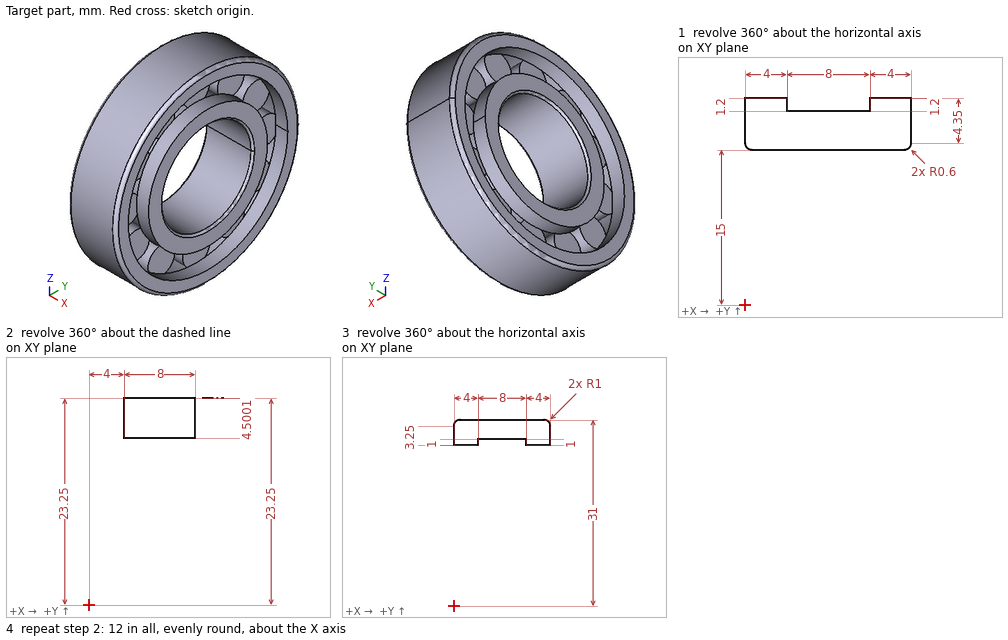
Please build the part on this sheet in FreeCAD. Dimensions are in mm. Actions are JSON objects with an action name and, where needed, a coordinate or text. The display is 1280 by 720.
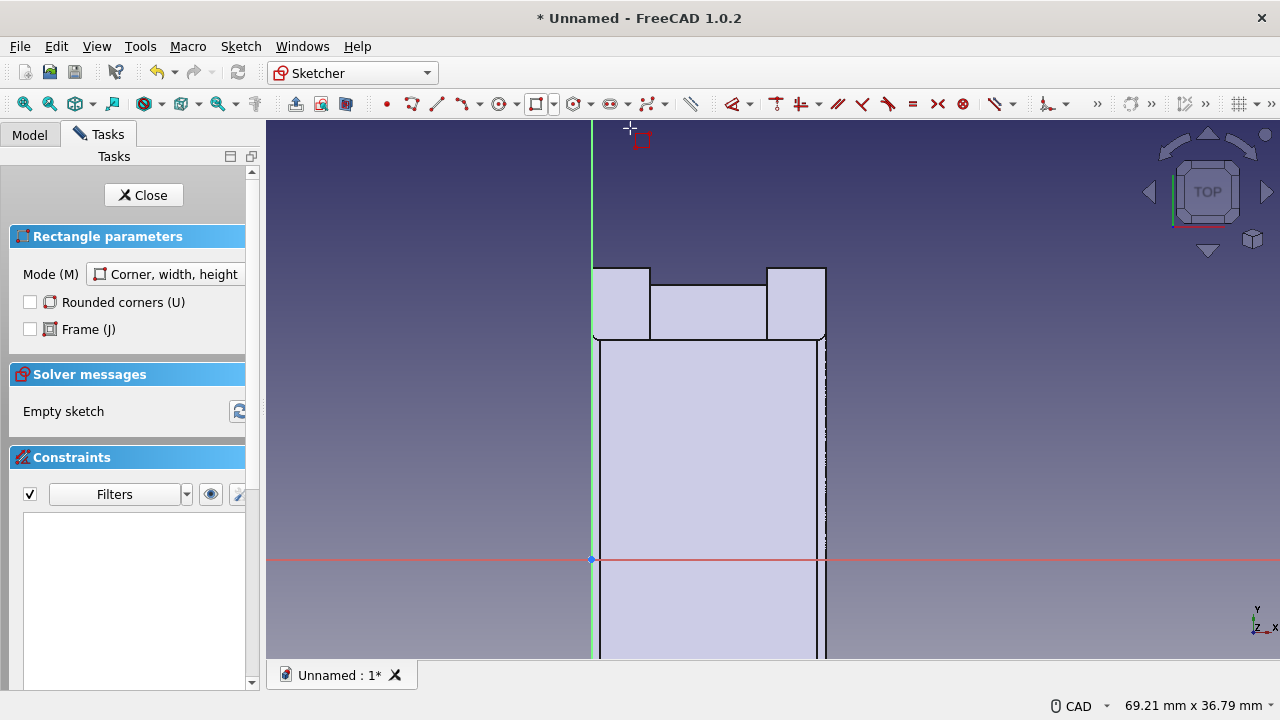
{"action": "left_click", "coordinate": [650, 219]}
{"action": "mouse_move", "coordinate": [767, 285]}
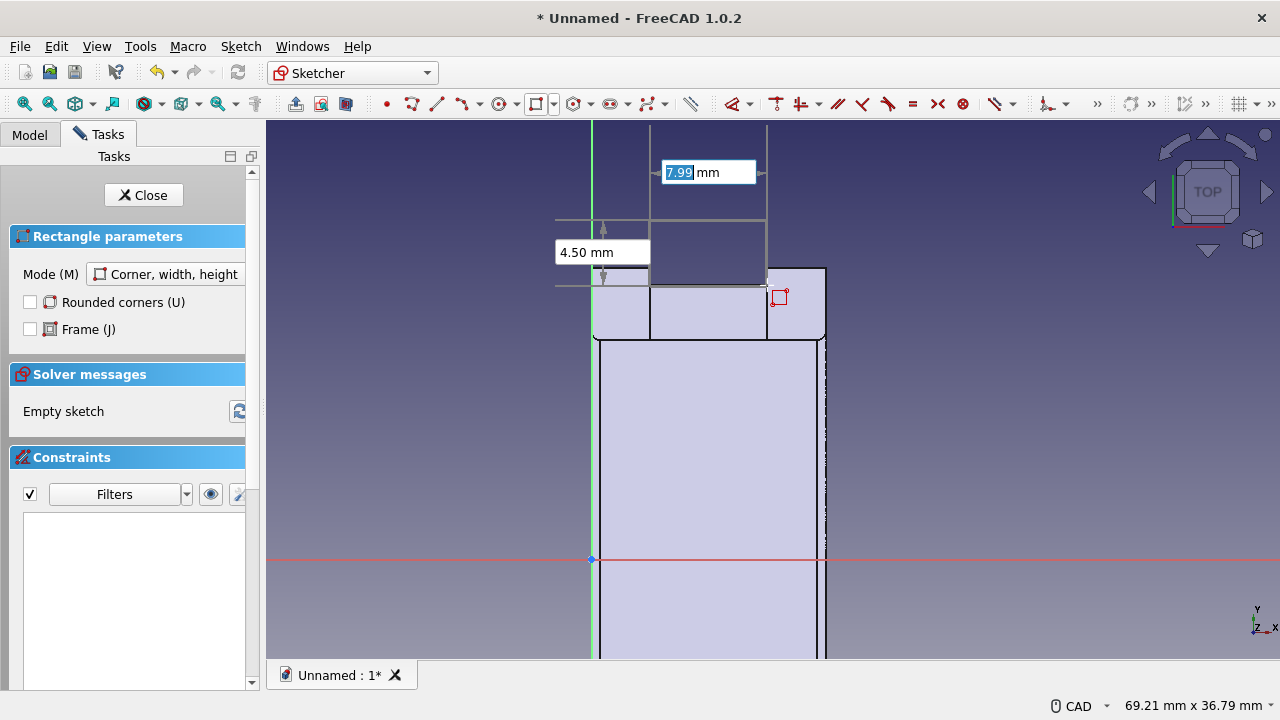
{"action": "type", "text": "8"}
{"action": "key", "text": "Tab"}
{"action": "type", "text": "4.5001"}
{"action": "key", "text": "Return"}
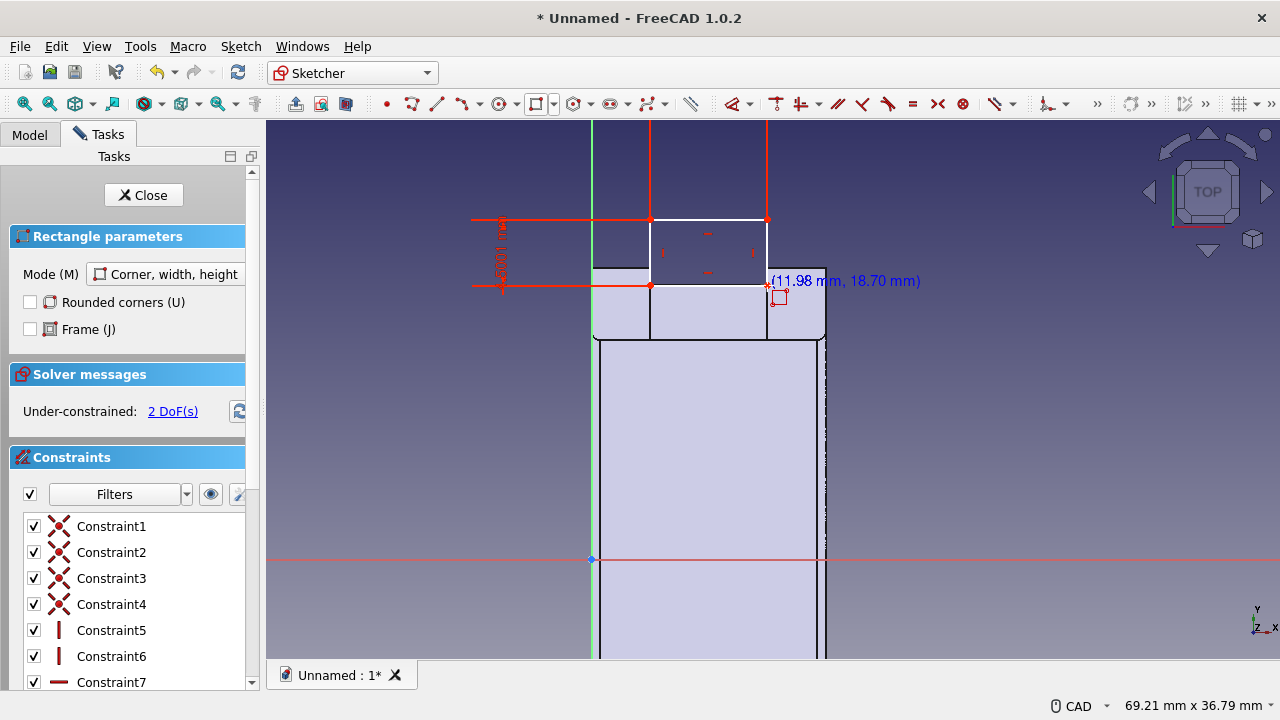
{"action": "left_click", "coordinate": [437, 104]}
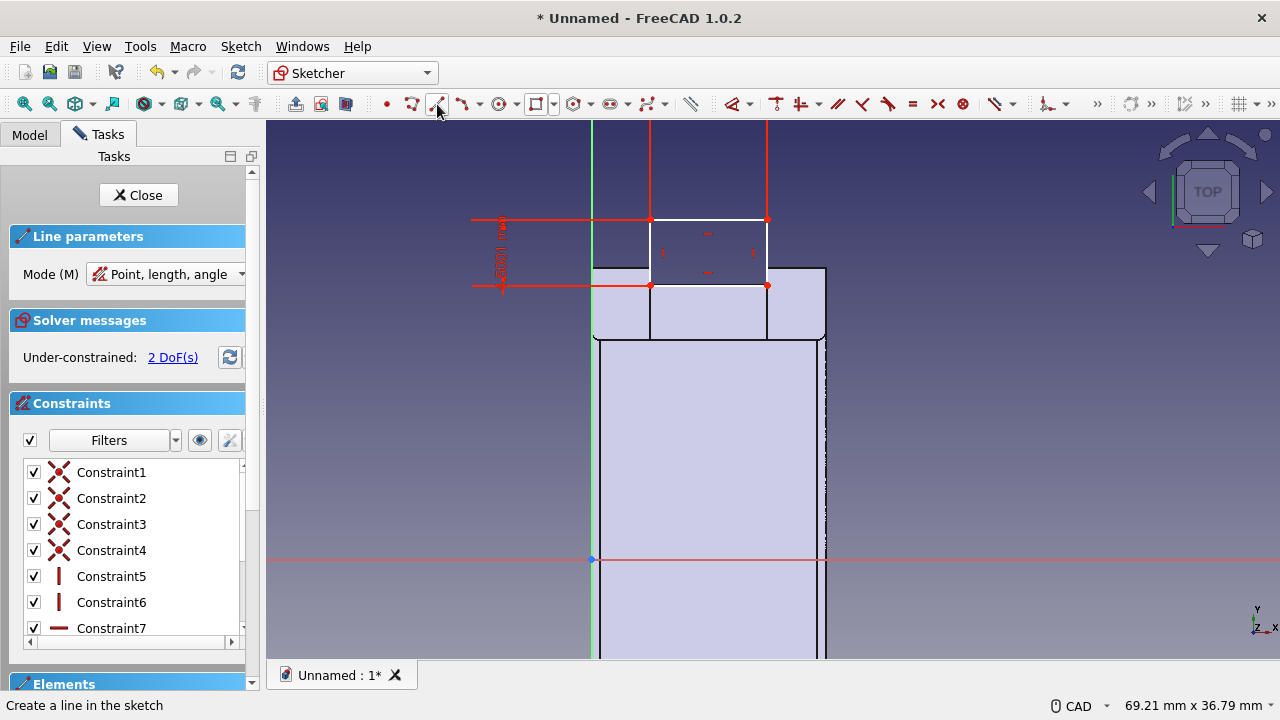
{"action": "scroll", "coordinate": [779, 219], "scroll_direction": "up", "scroll_amount": 2}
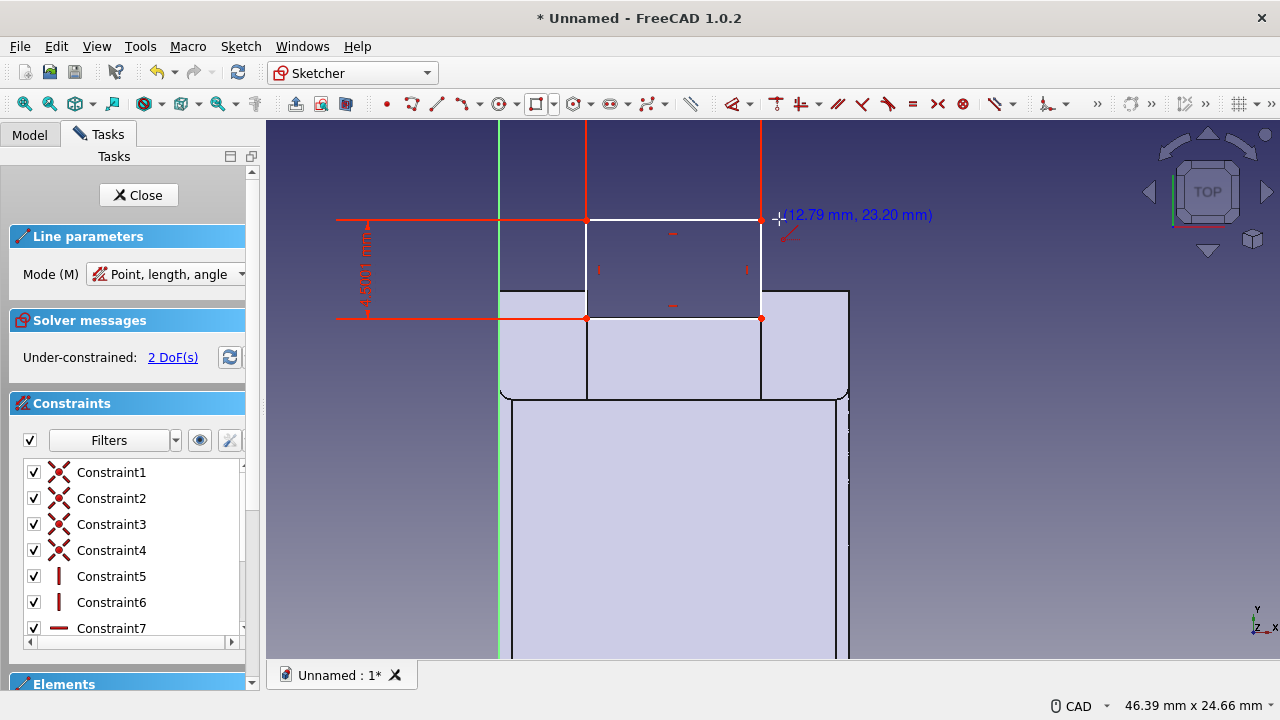
{"action": "left_click", "coordinate": [779, 219]}
{"action": "left_click", "coordinate": [831, 219]}
{"action": "key", "text": "Escape"}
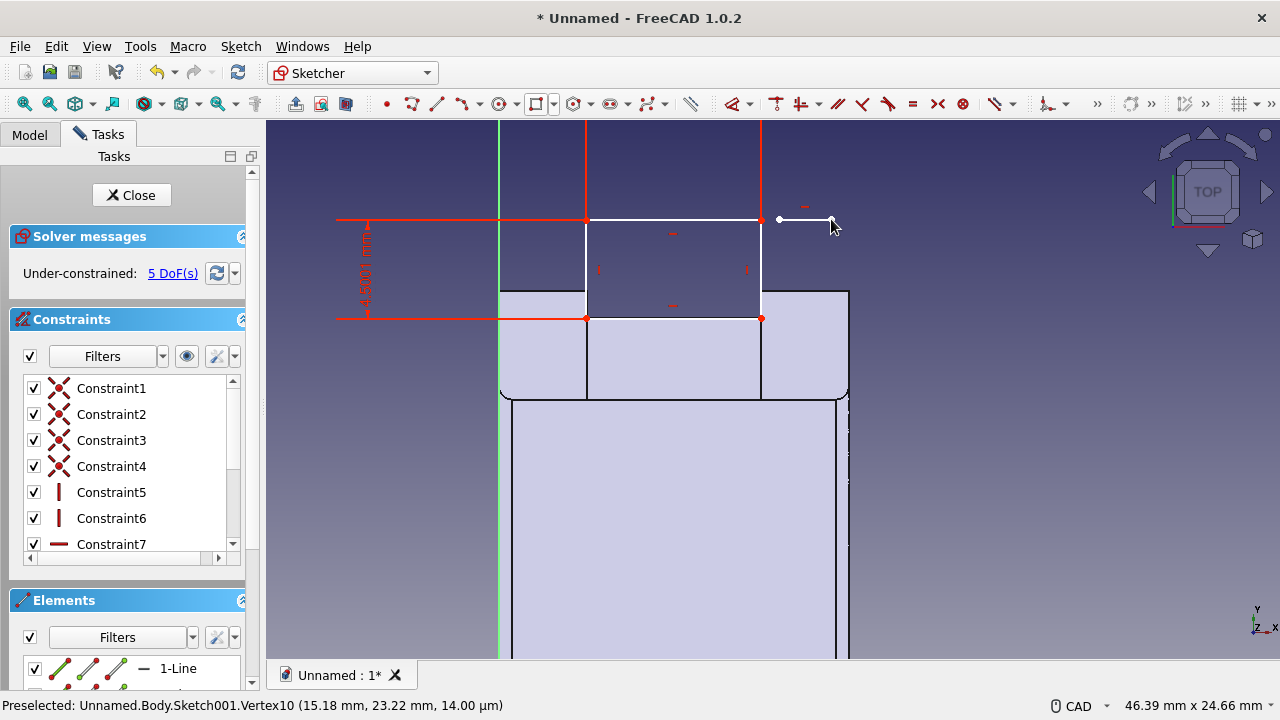
{"action": "left_click", "coordinate": [795, 220]}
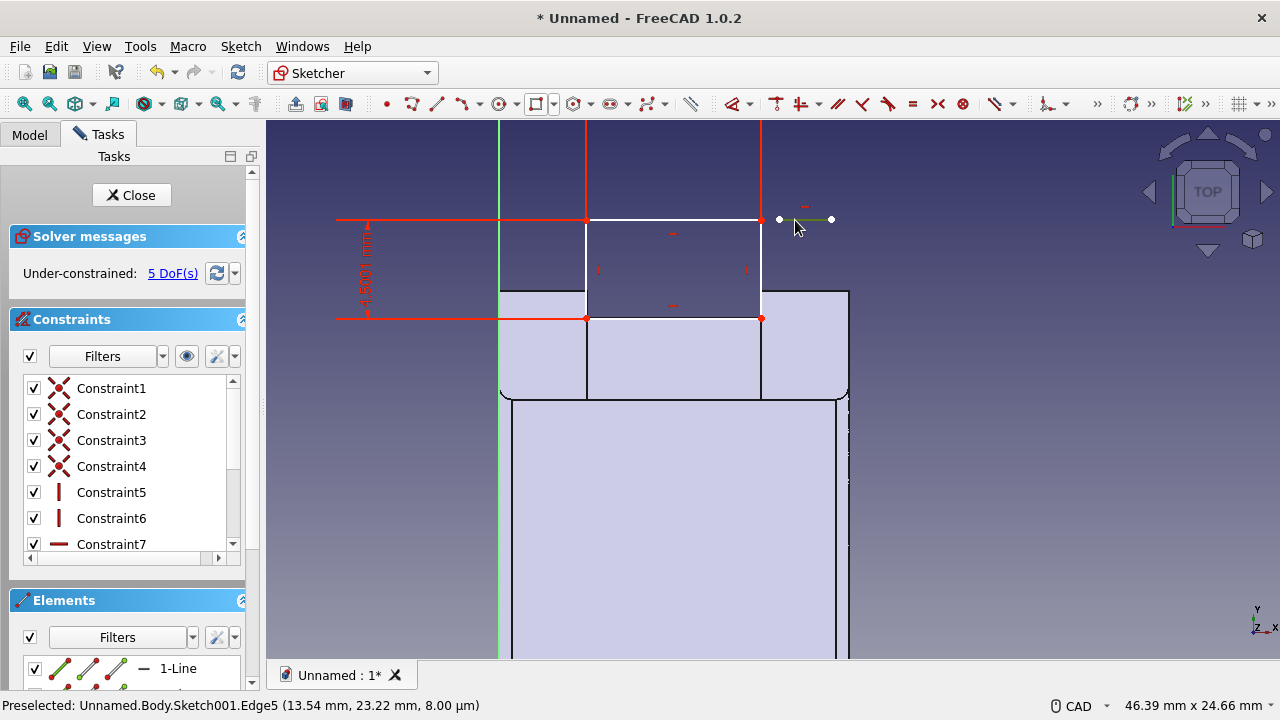
{"action": "left_click", "coordinate": [691, 104]}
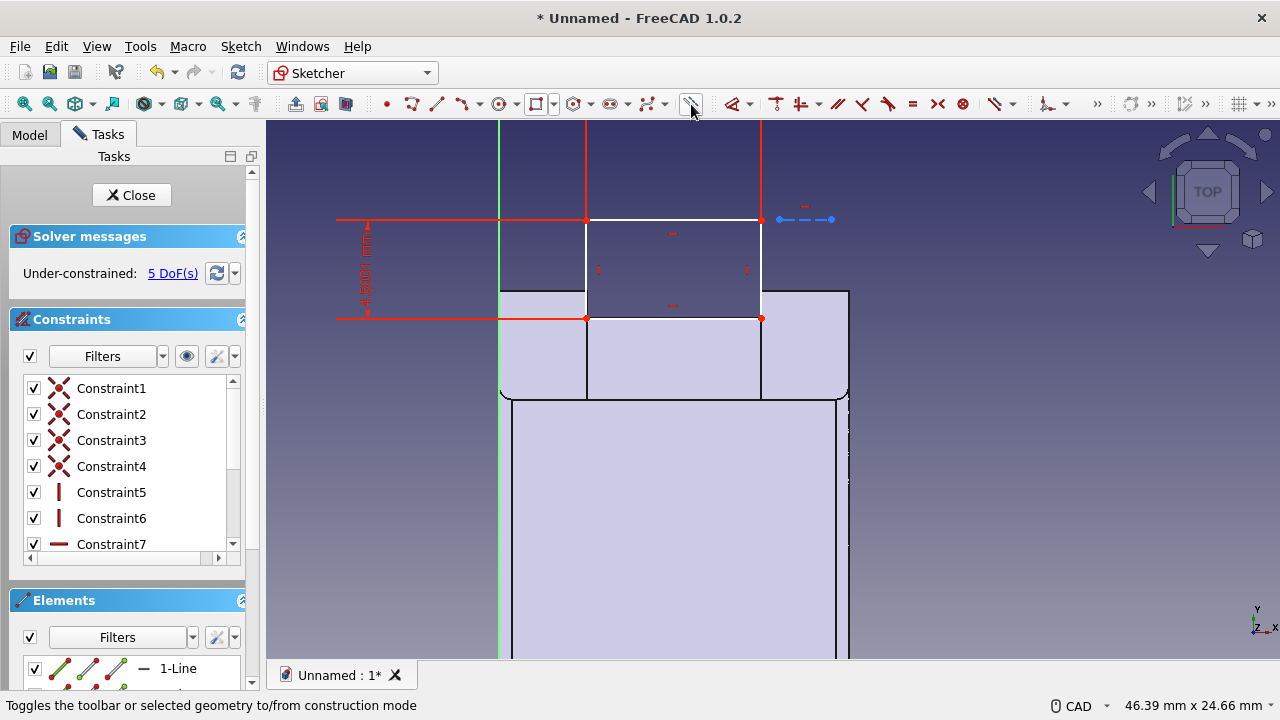
{"action": "key", "text": "d"}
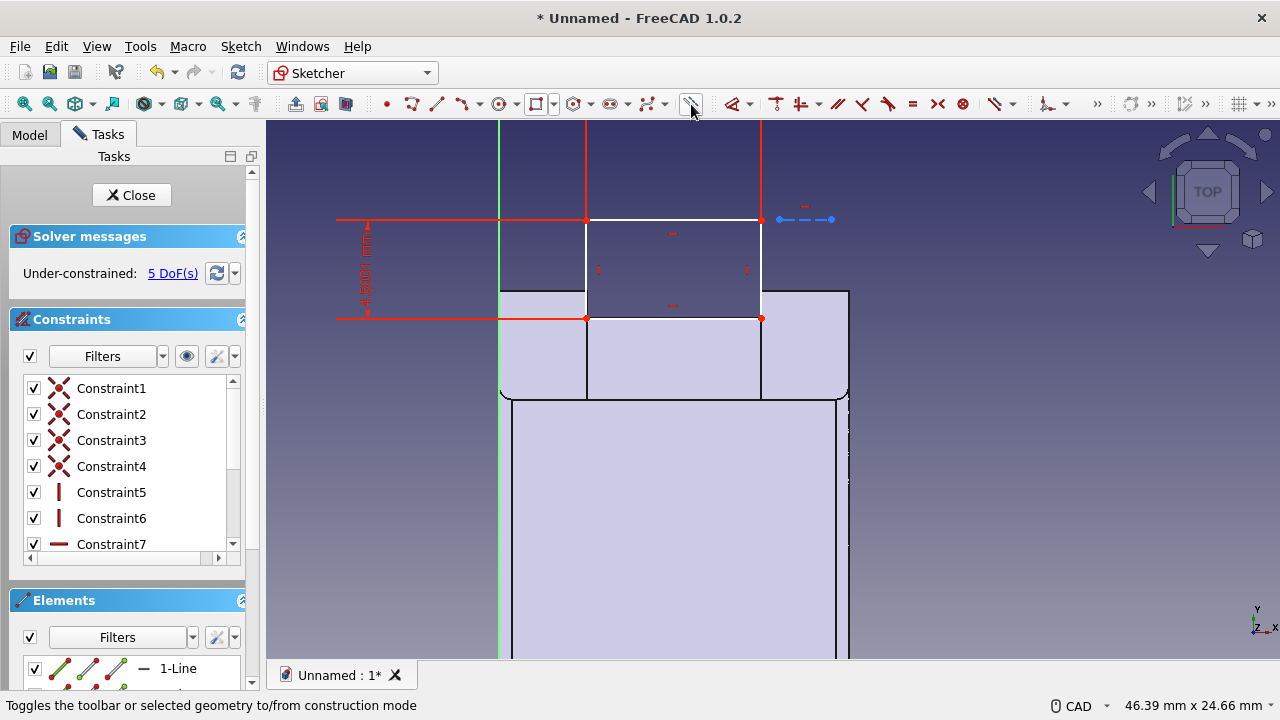
{"action": "left_click", "coordinate": [586, 220]}
{"action": "left_click", "coordinate": [543, 186]}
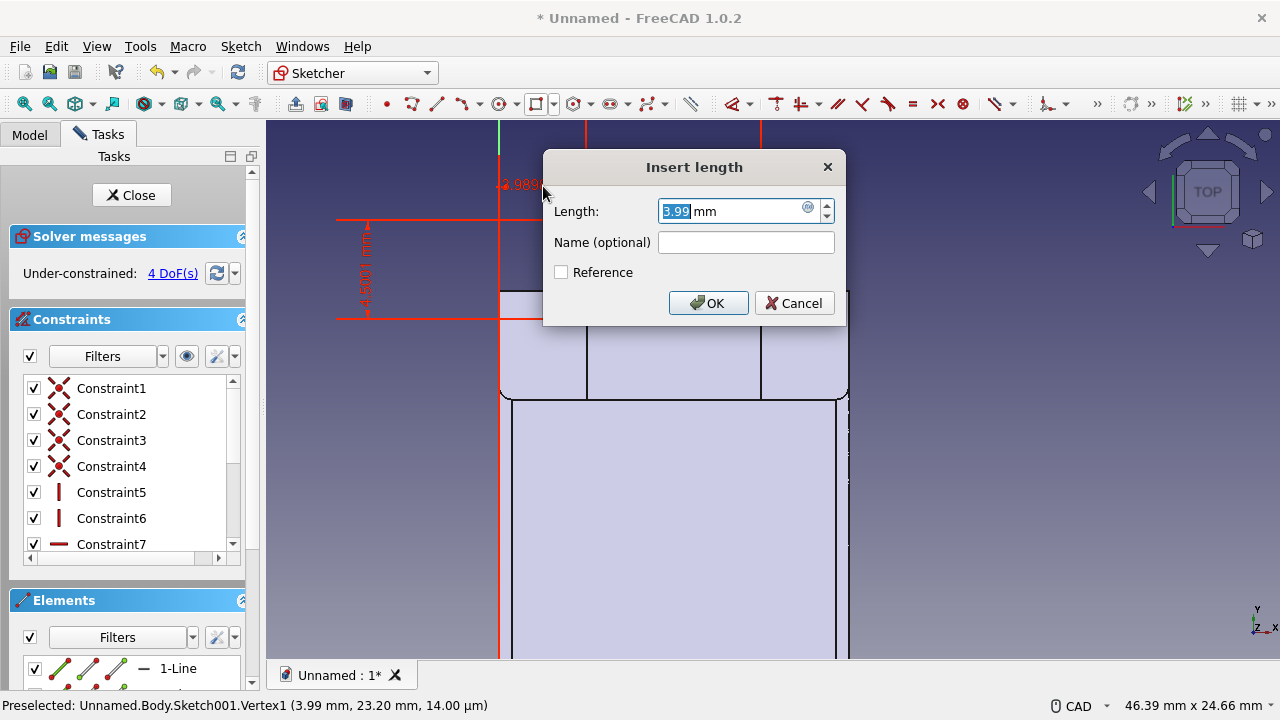
{"action": "type", "text": "4"}
{"action": "key", "text": "Return"}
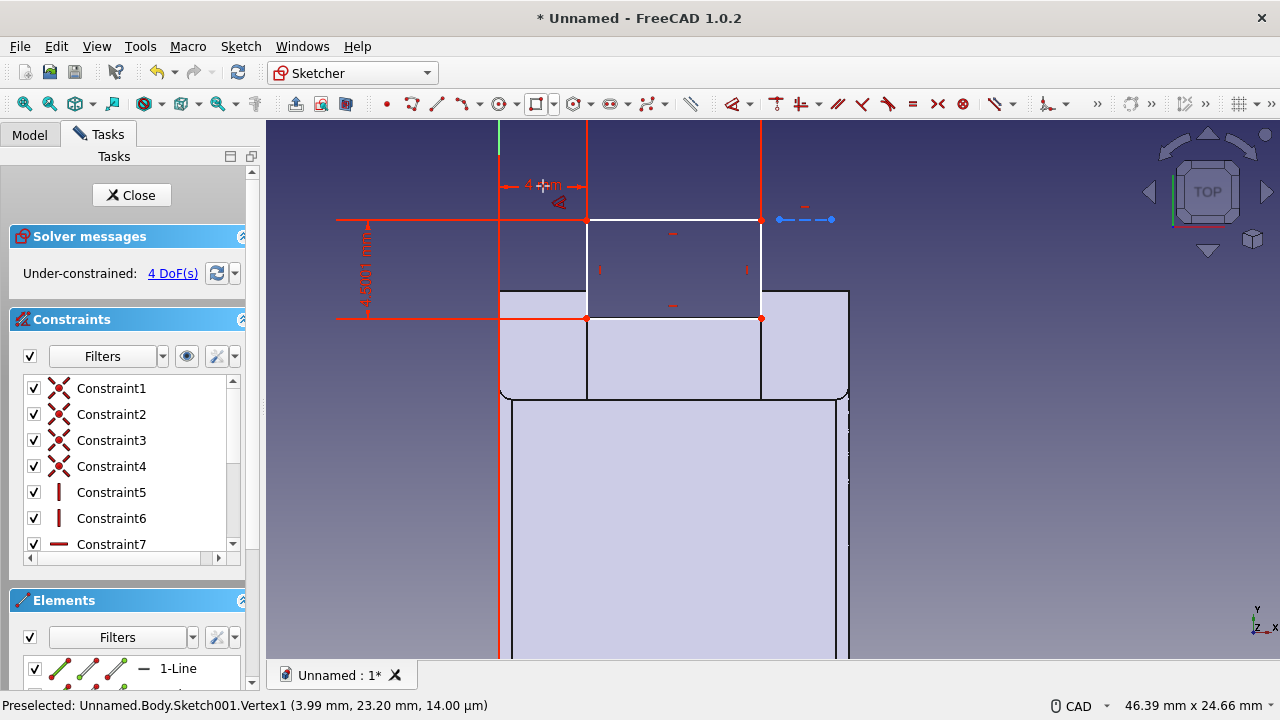
{"action": "left_click", "coordinate": [587, 220]}
{"action": "left_click", "coordinate": [465, 426]}